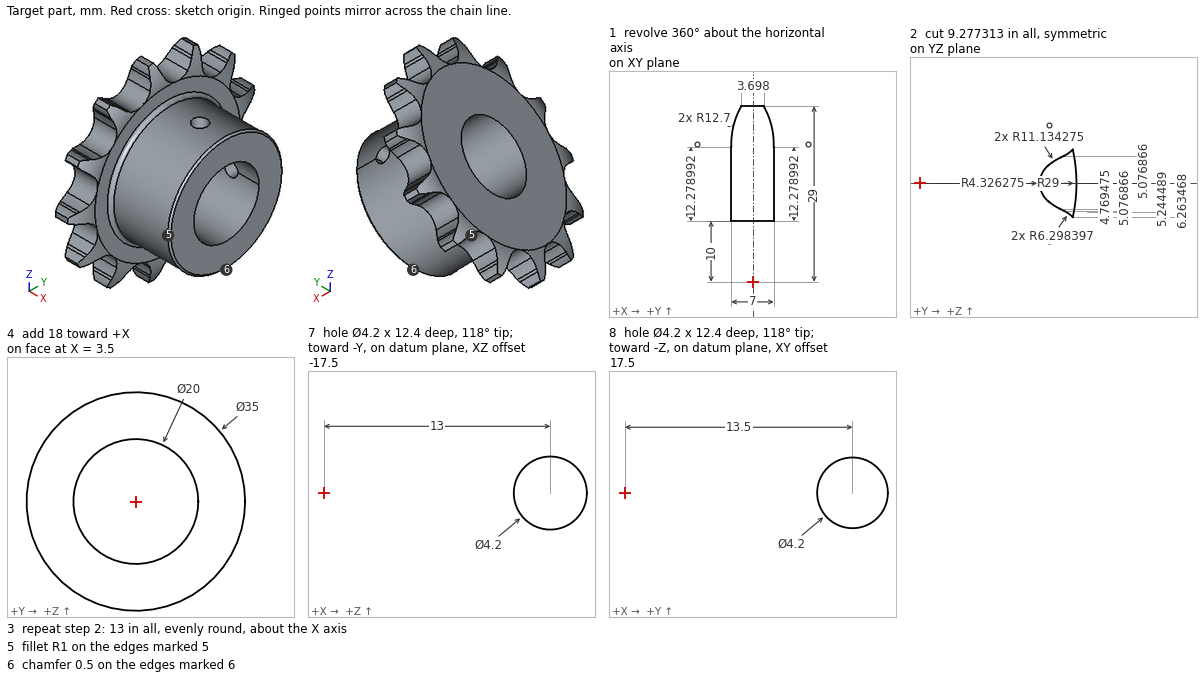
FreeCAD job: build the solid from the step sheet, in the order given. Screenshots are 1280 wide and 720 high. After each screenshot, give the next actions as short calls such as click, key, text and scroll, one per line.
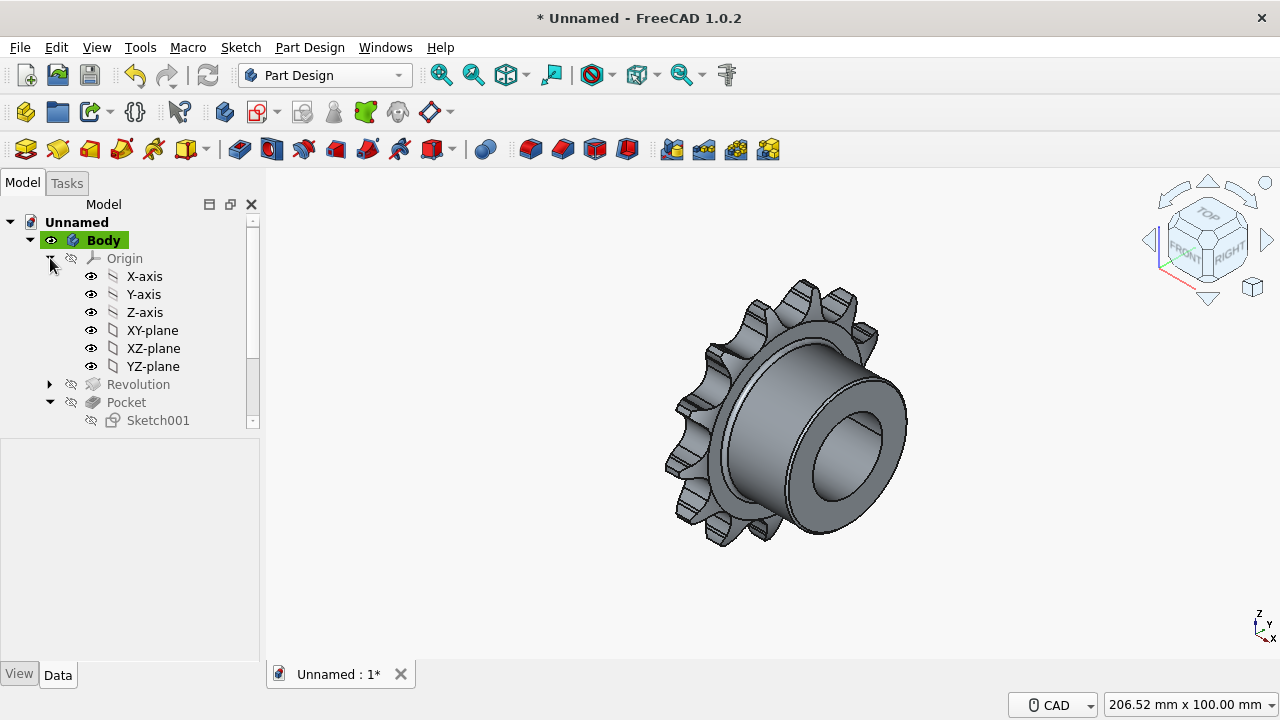
click(136, 348)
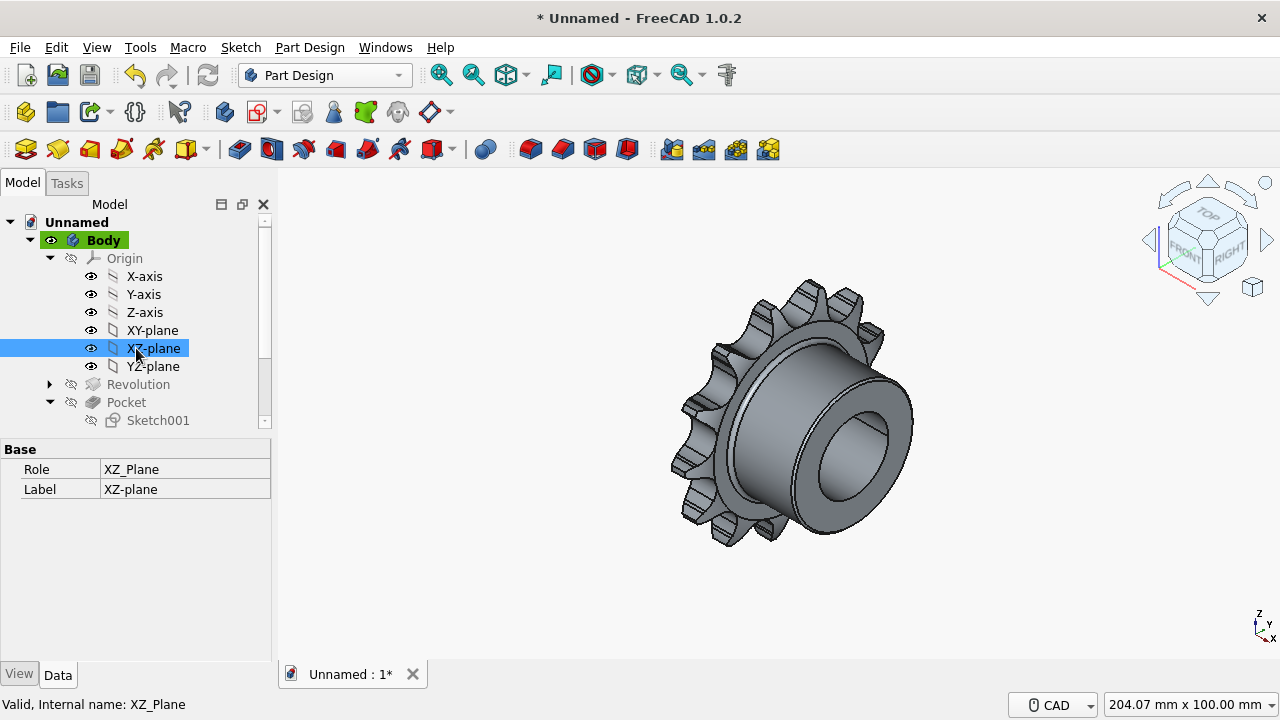
click(430, 112)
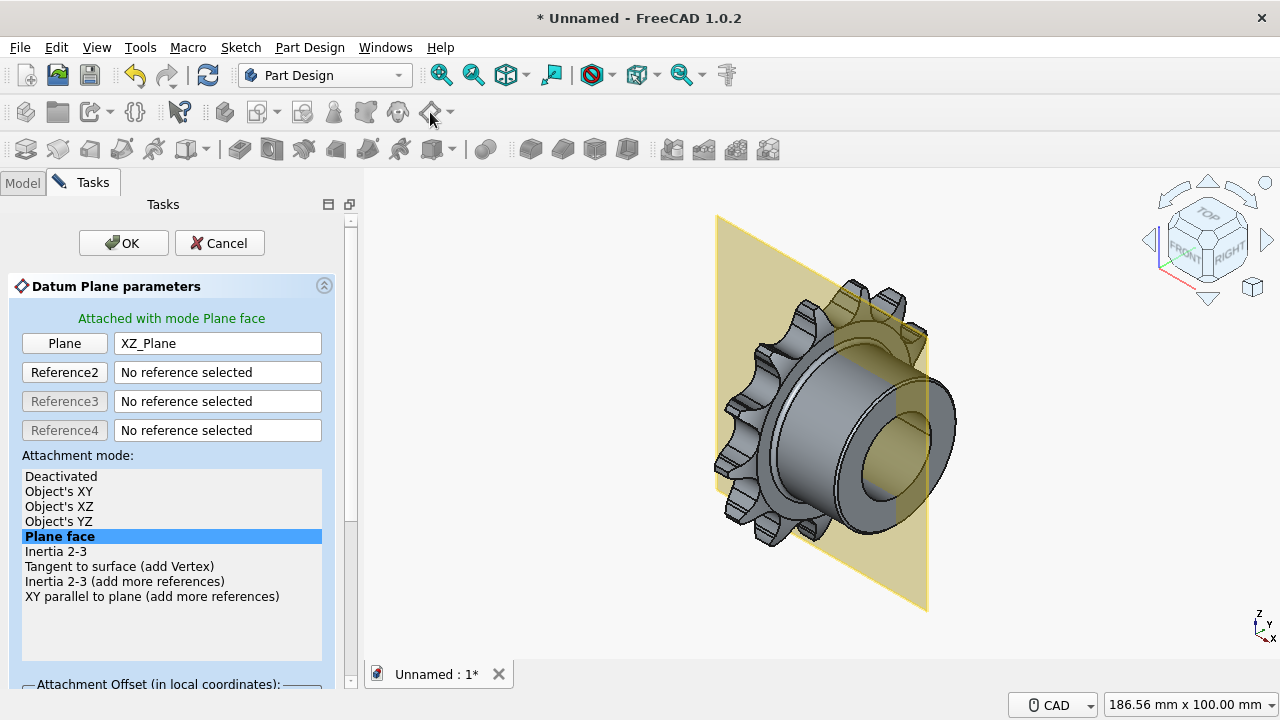
scroll(351, 451, down, 3)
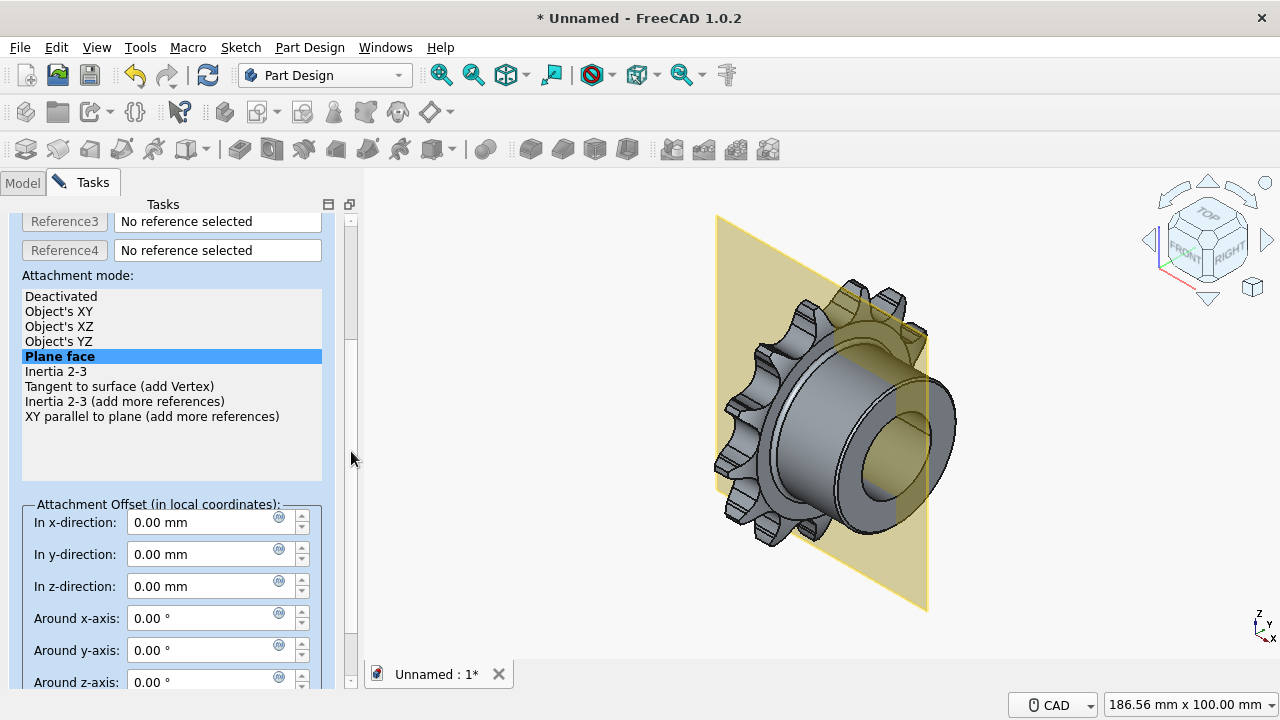
triple_click(210, 586)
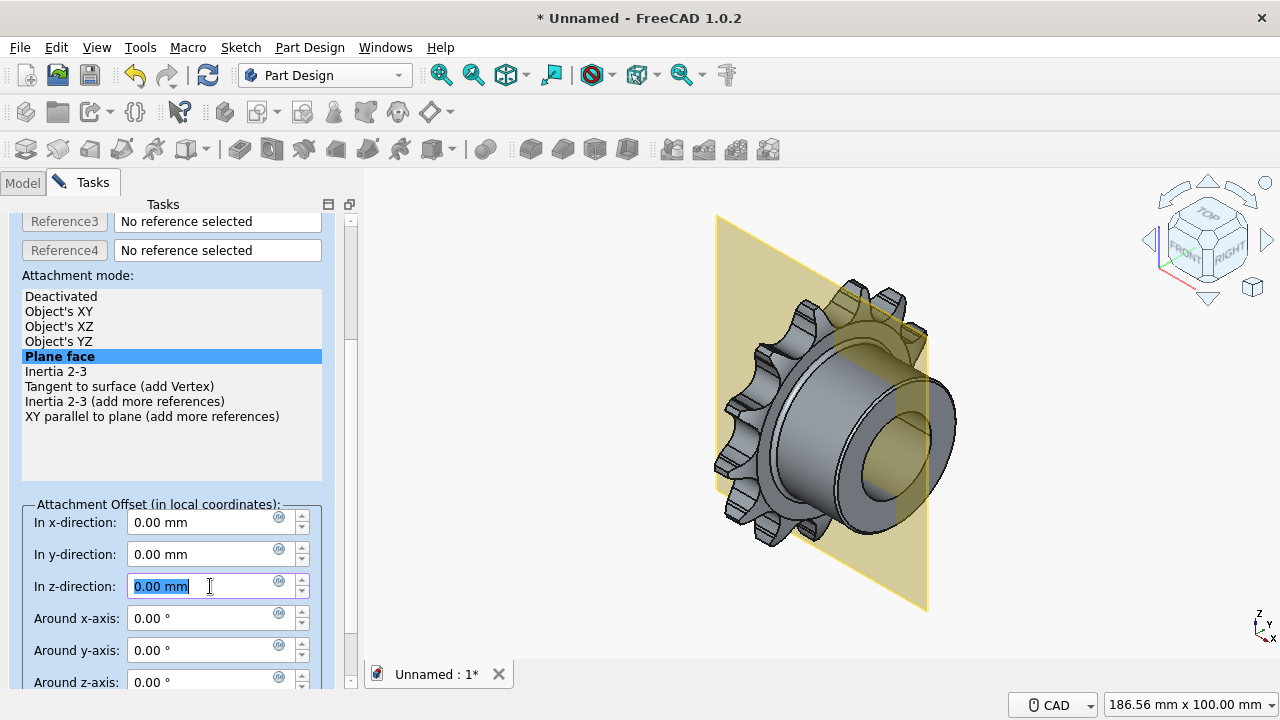
text(-17.5)
key(Tab)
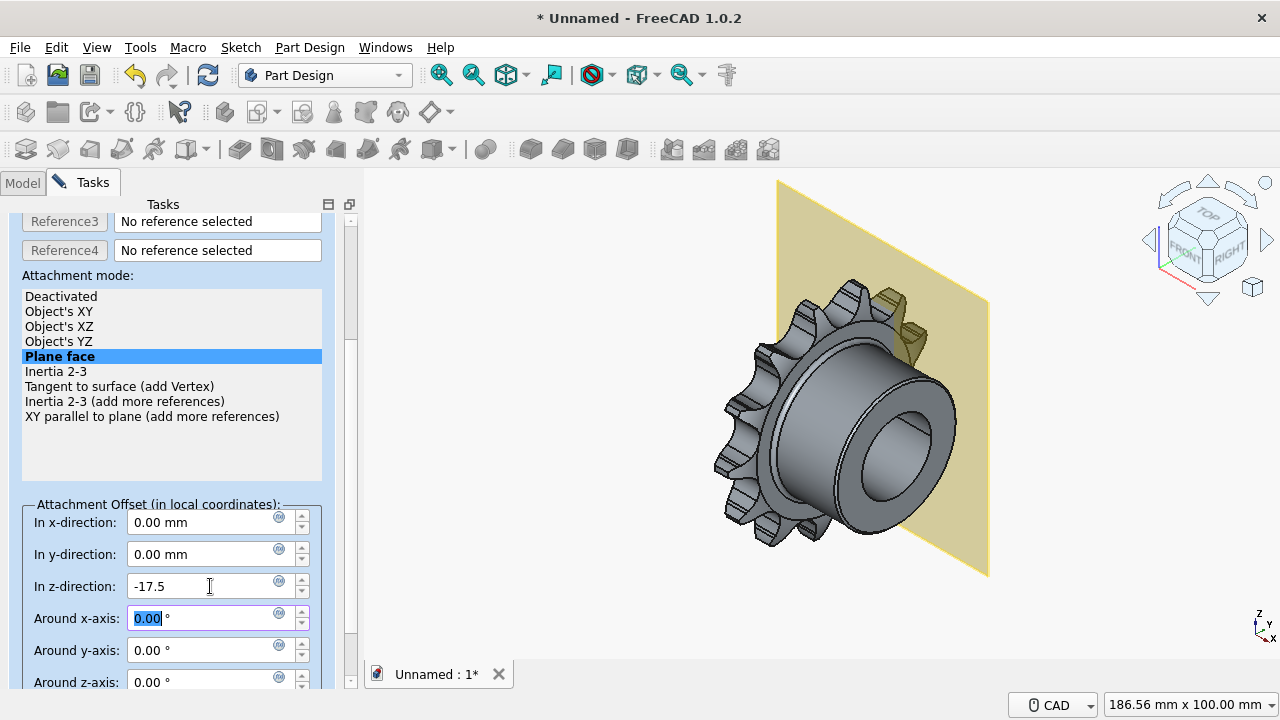
scroll(351, 451, up, 4)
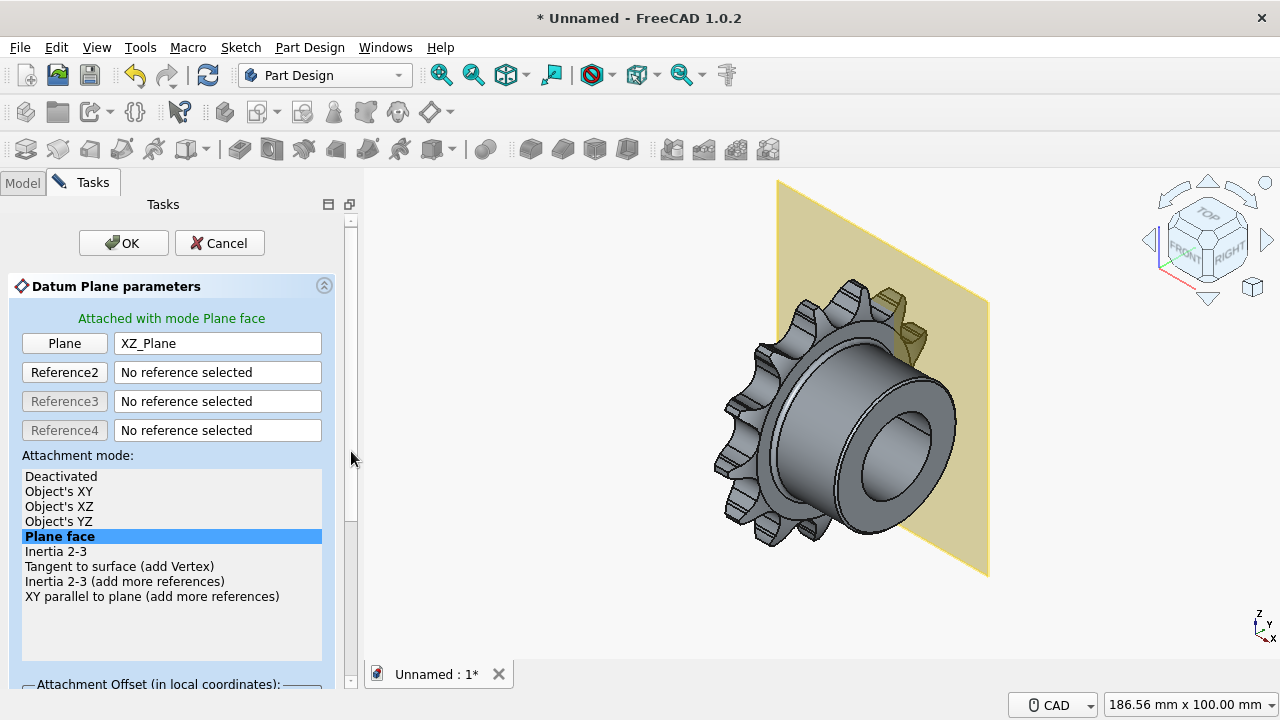
click(124, 243)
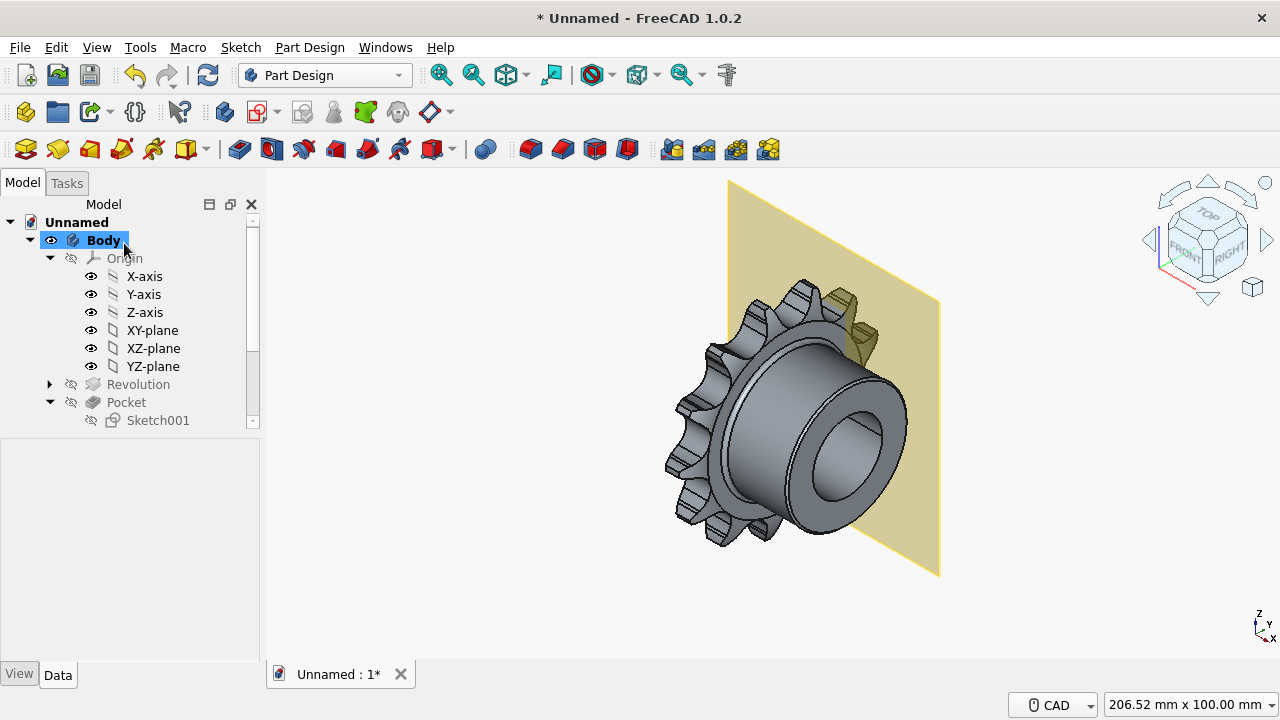
scroll(100, 326, down, 3)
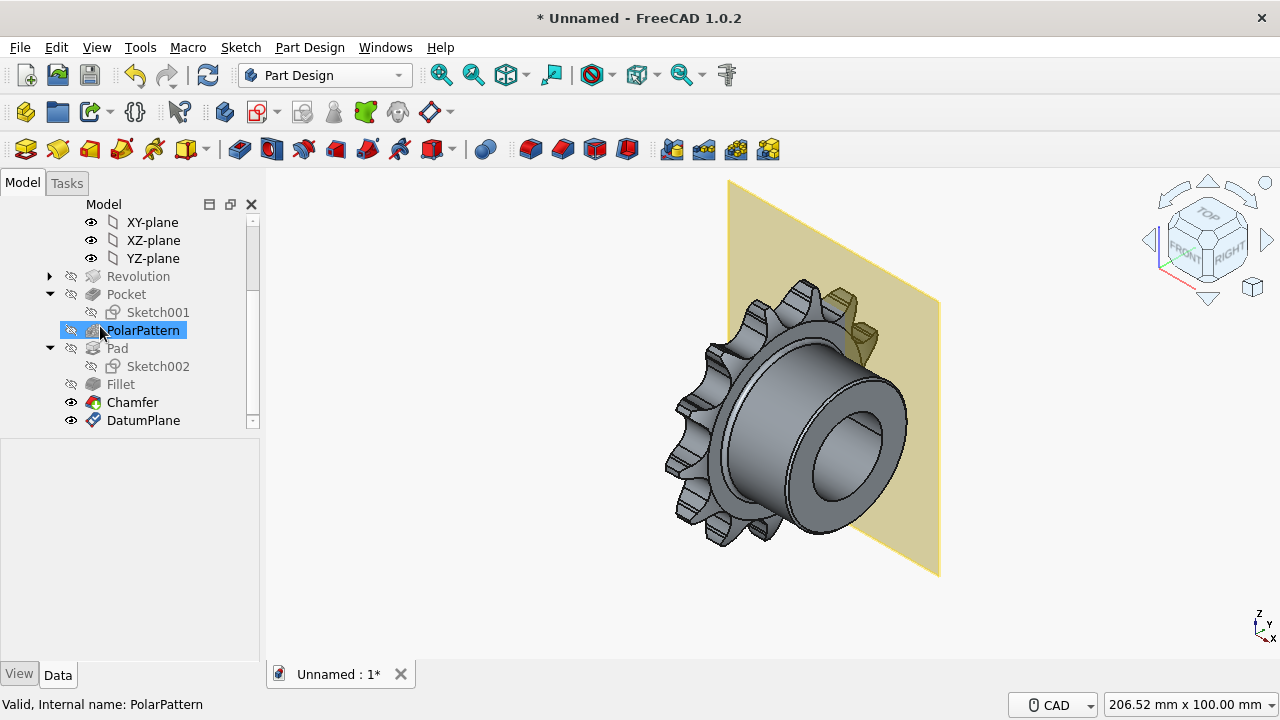
click(116, 420)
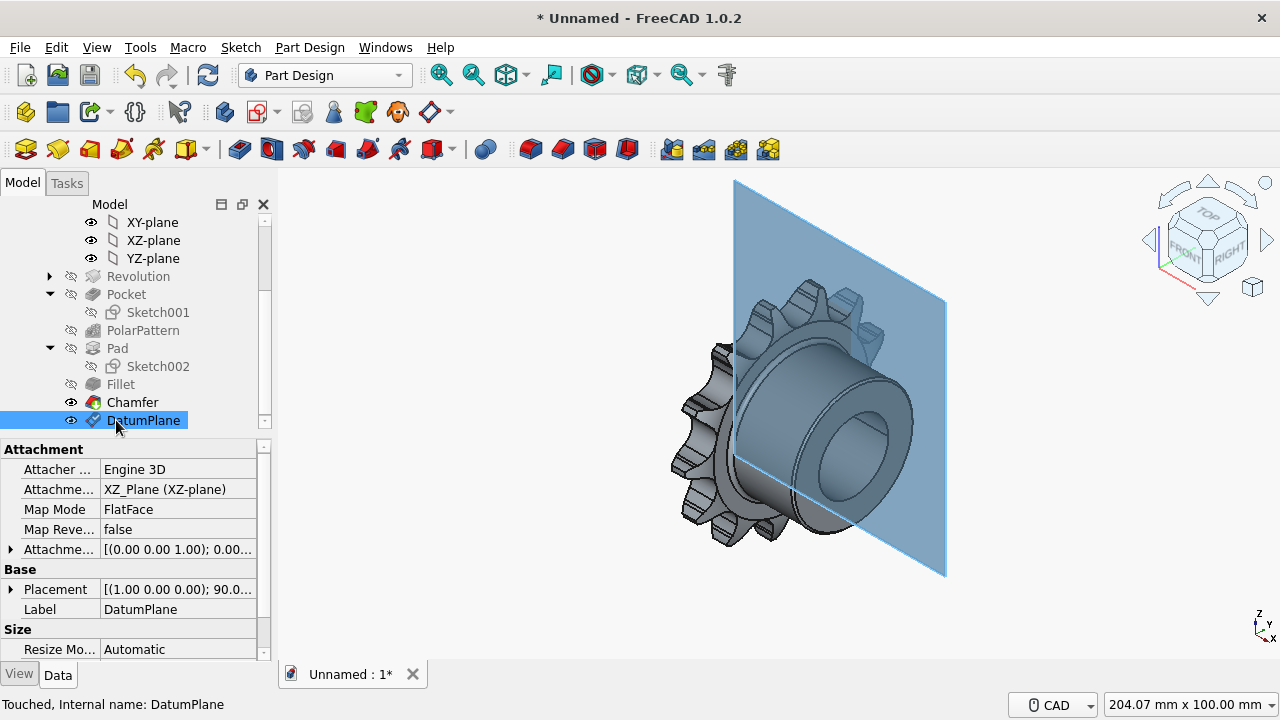
click(258, 112)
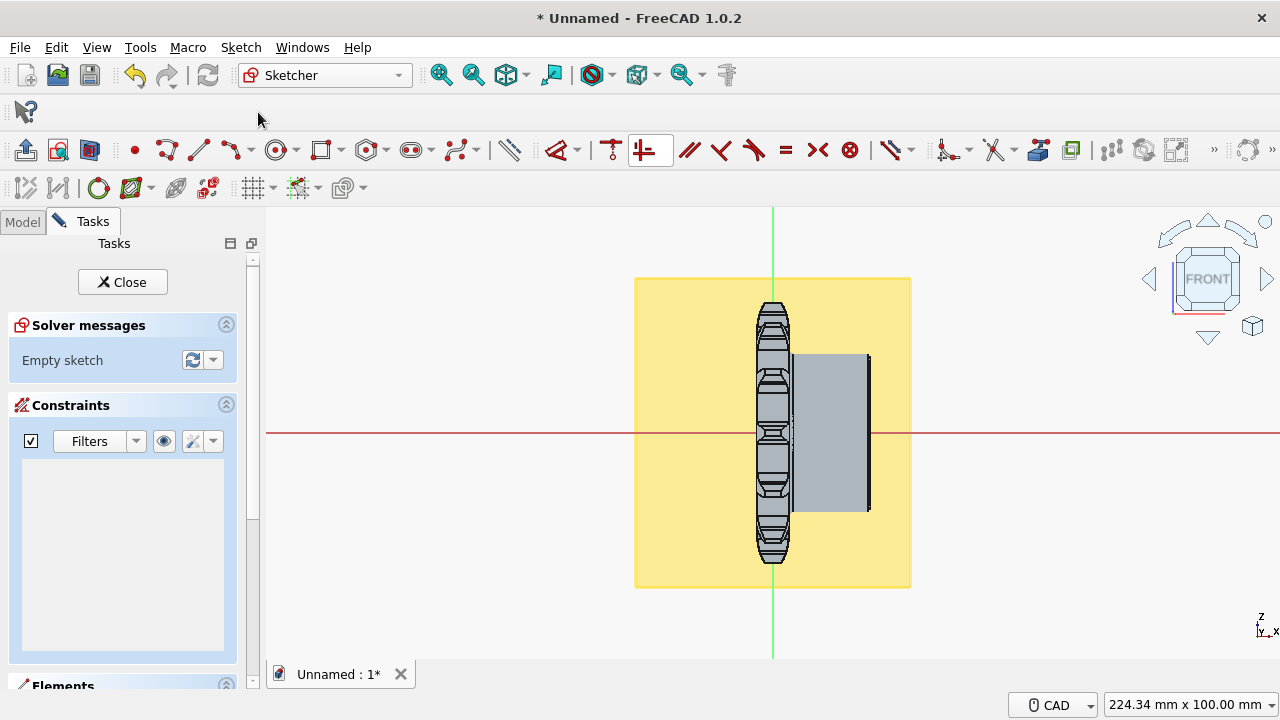
click(90, 150)